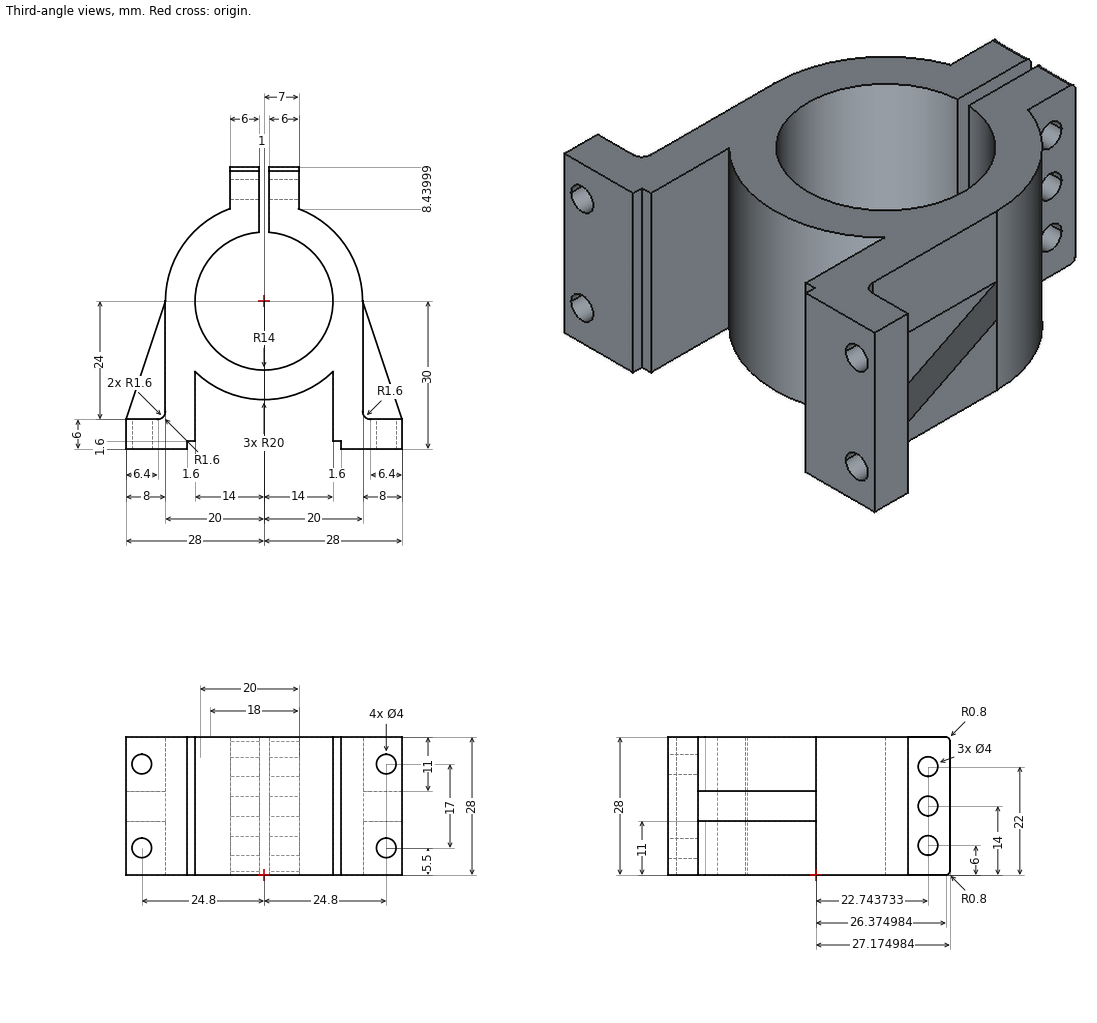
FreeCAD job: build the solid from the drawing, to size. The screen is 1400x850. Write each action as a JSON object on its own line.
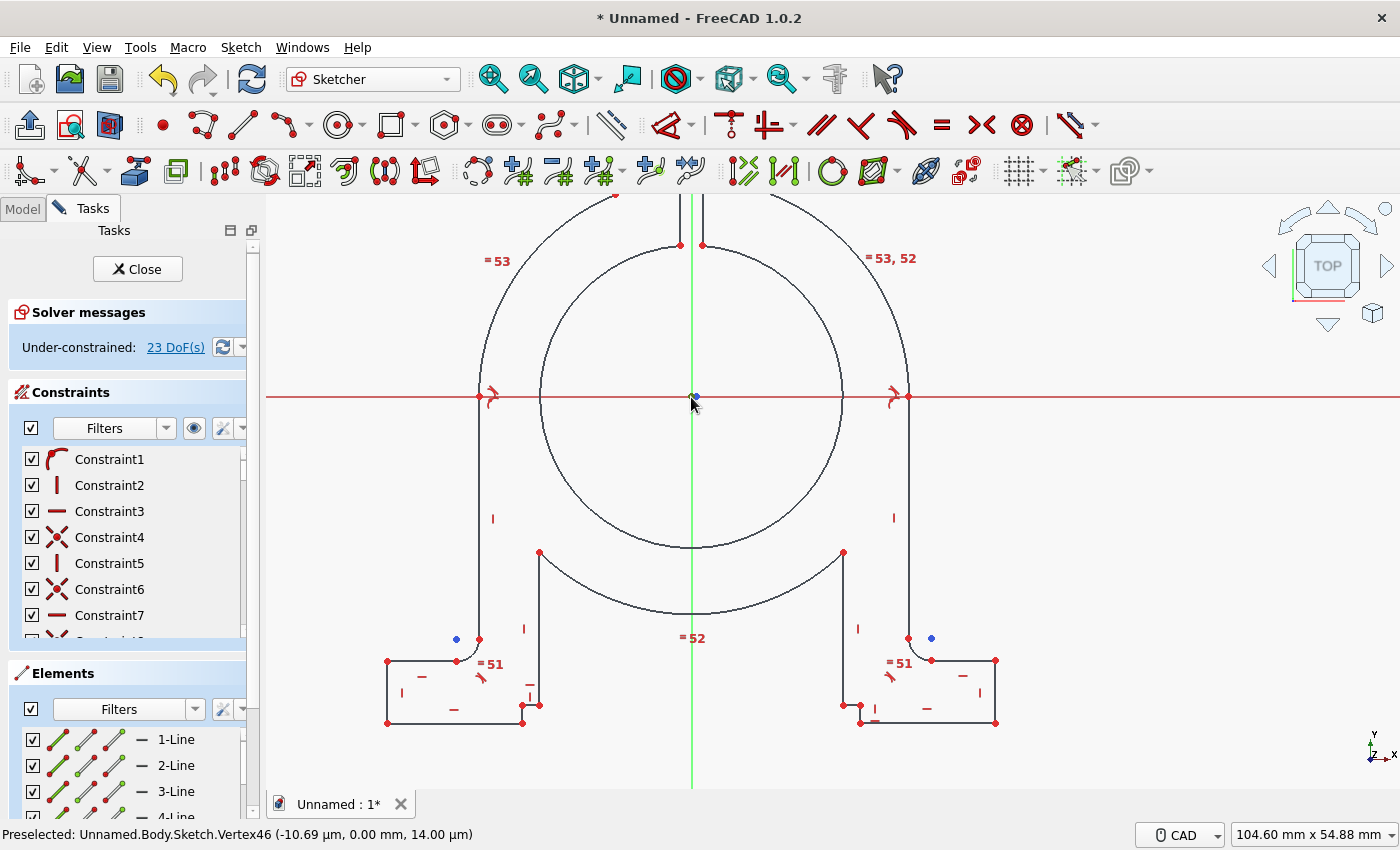
{"action": "left_click", "coordinate": [692, 722]}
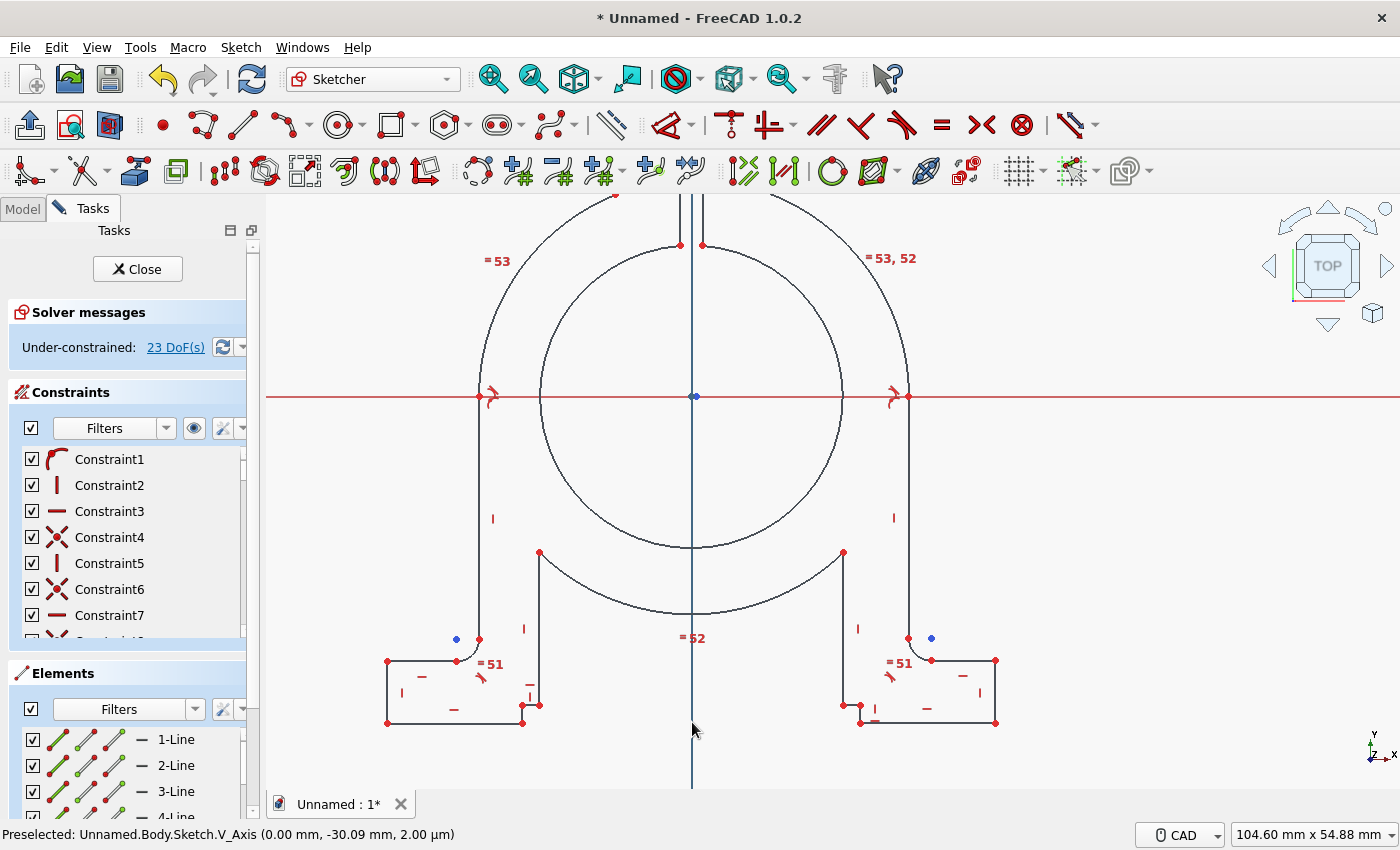
{"action": "left_click", "coordinate": [730, 126]}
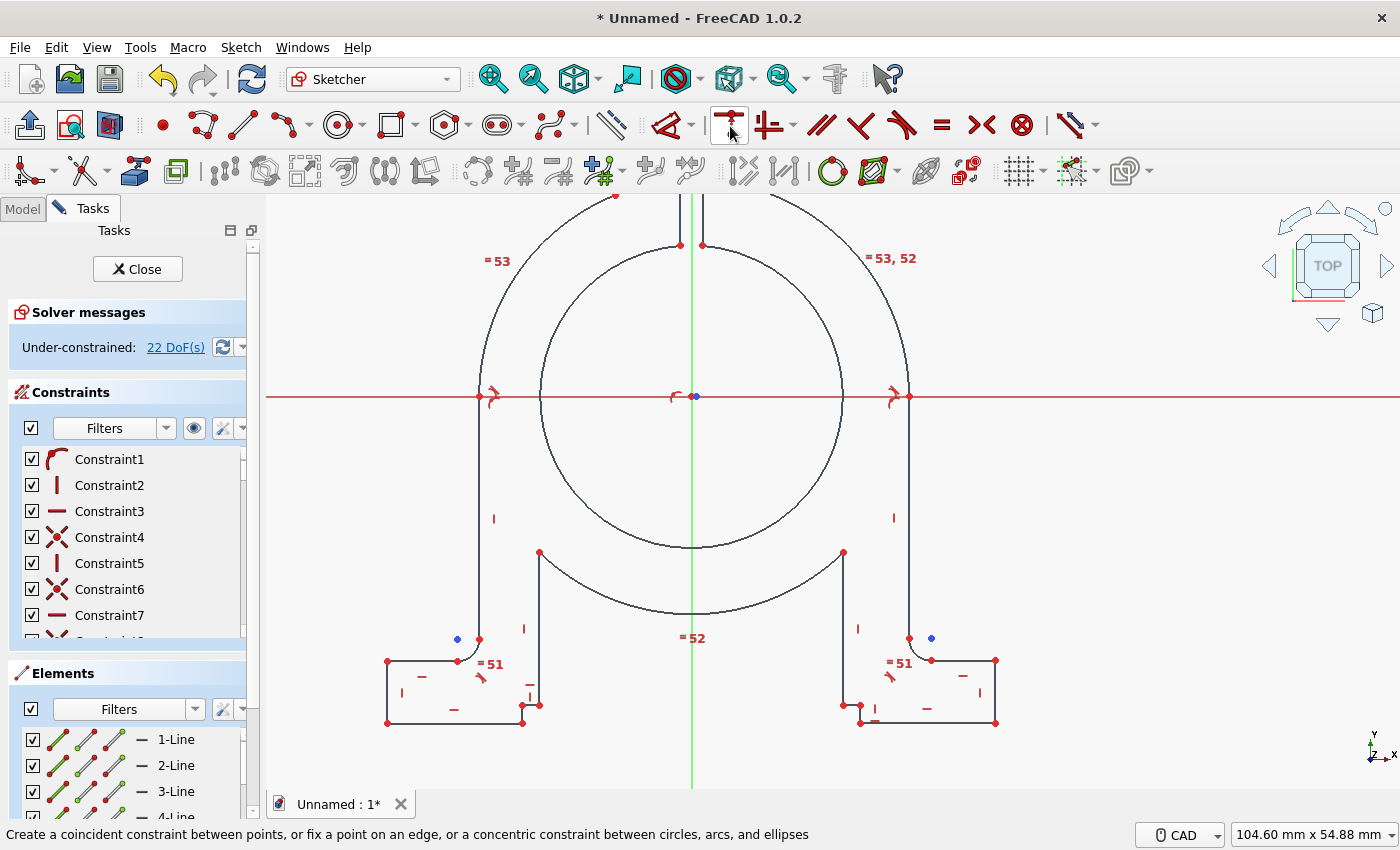
{"action": "left_click", "coordinate": [697, 397]}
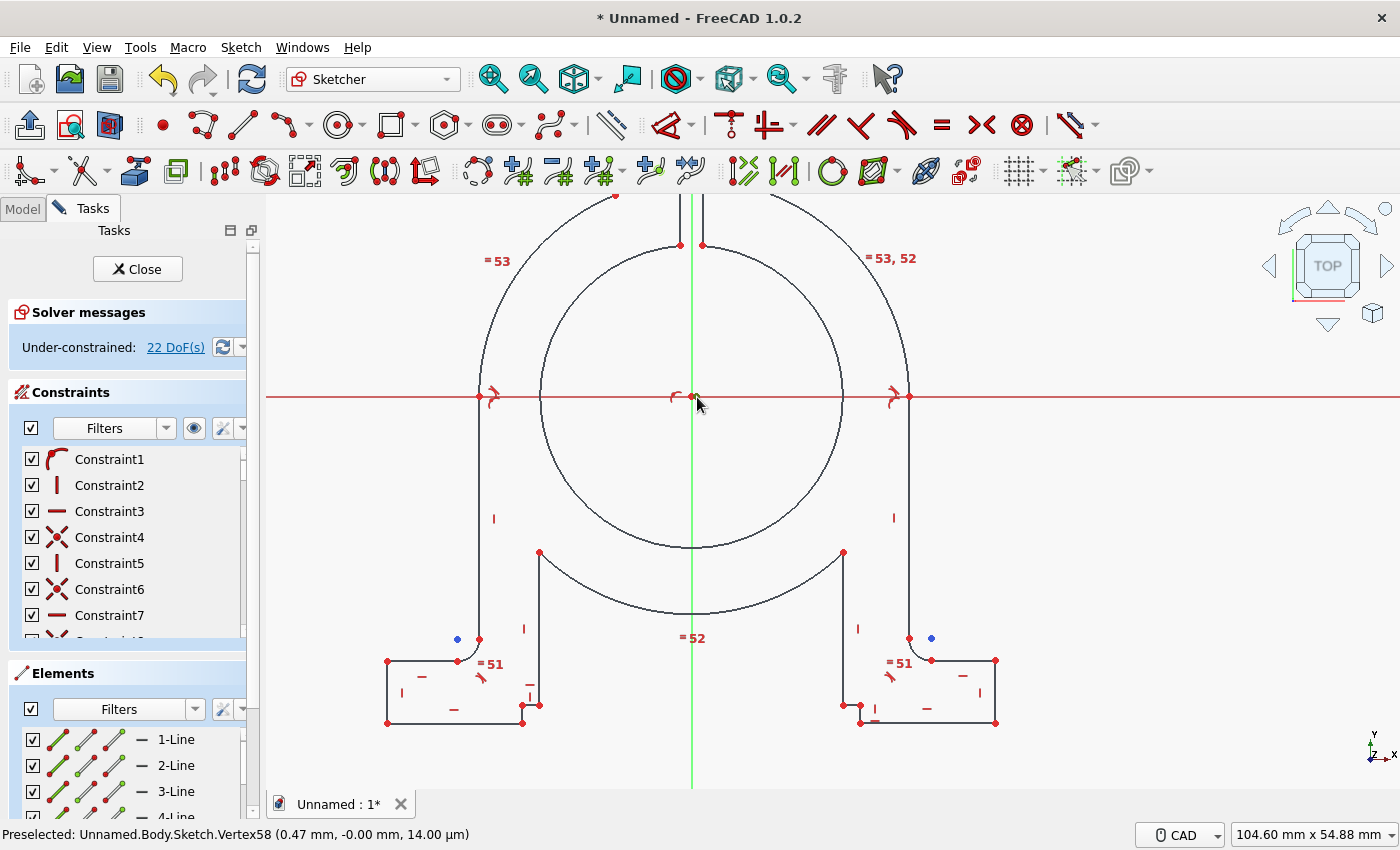
{"action": "left_click", "coordinate": [692, 722]}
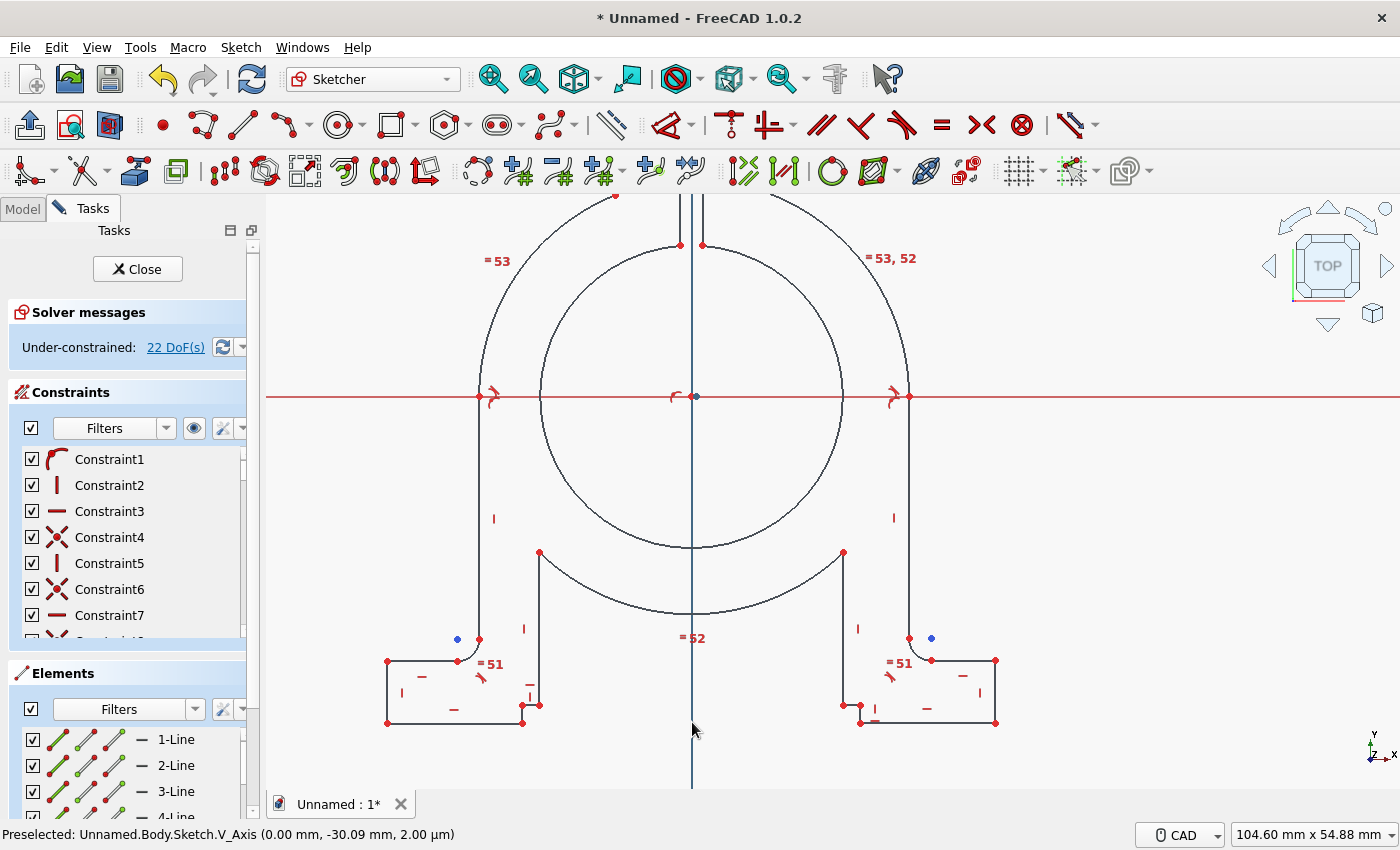
{"action": "left_click", "coordinate": [730, 126]}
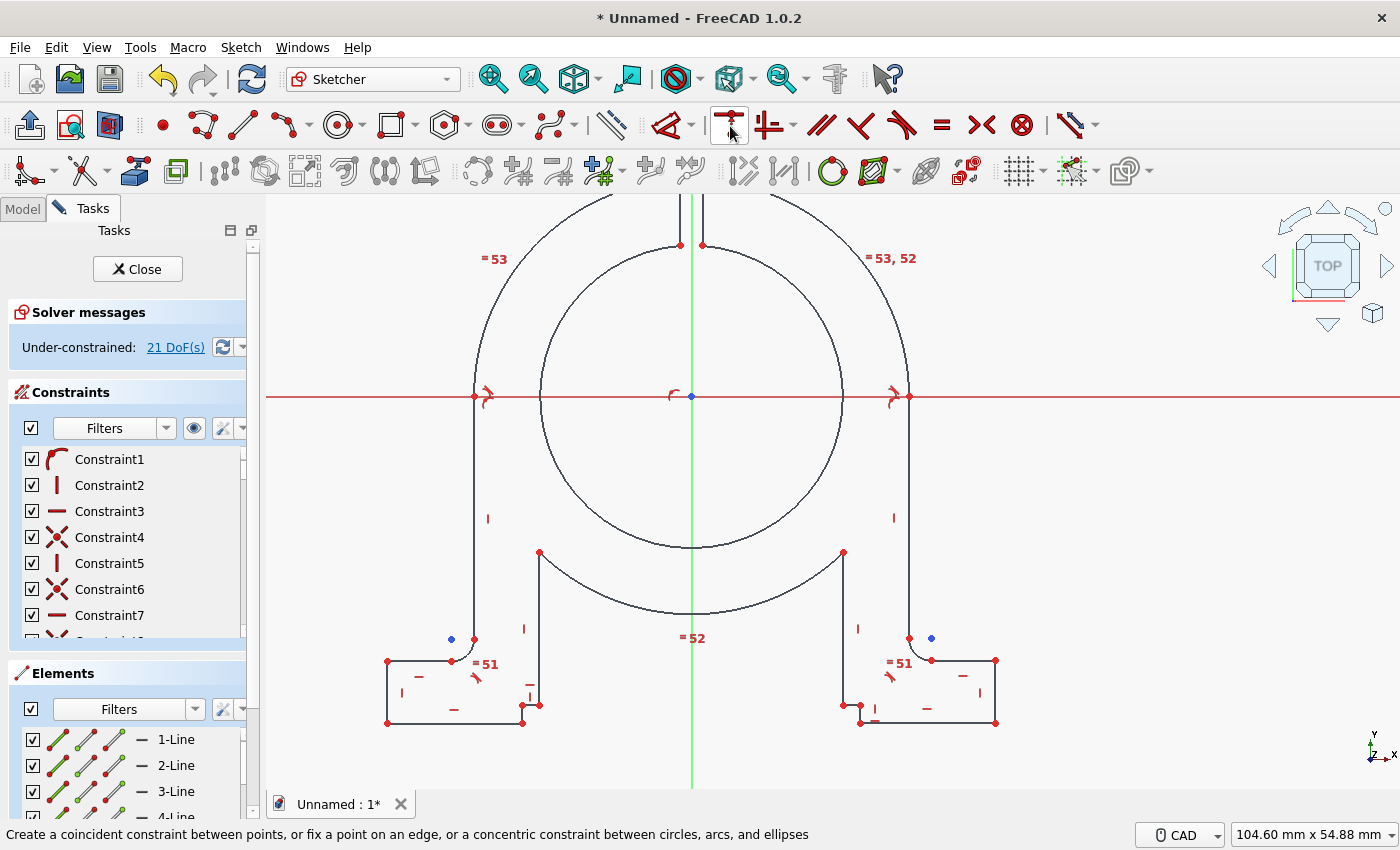
{"action": "left_click", "coordinate": [666, 126]}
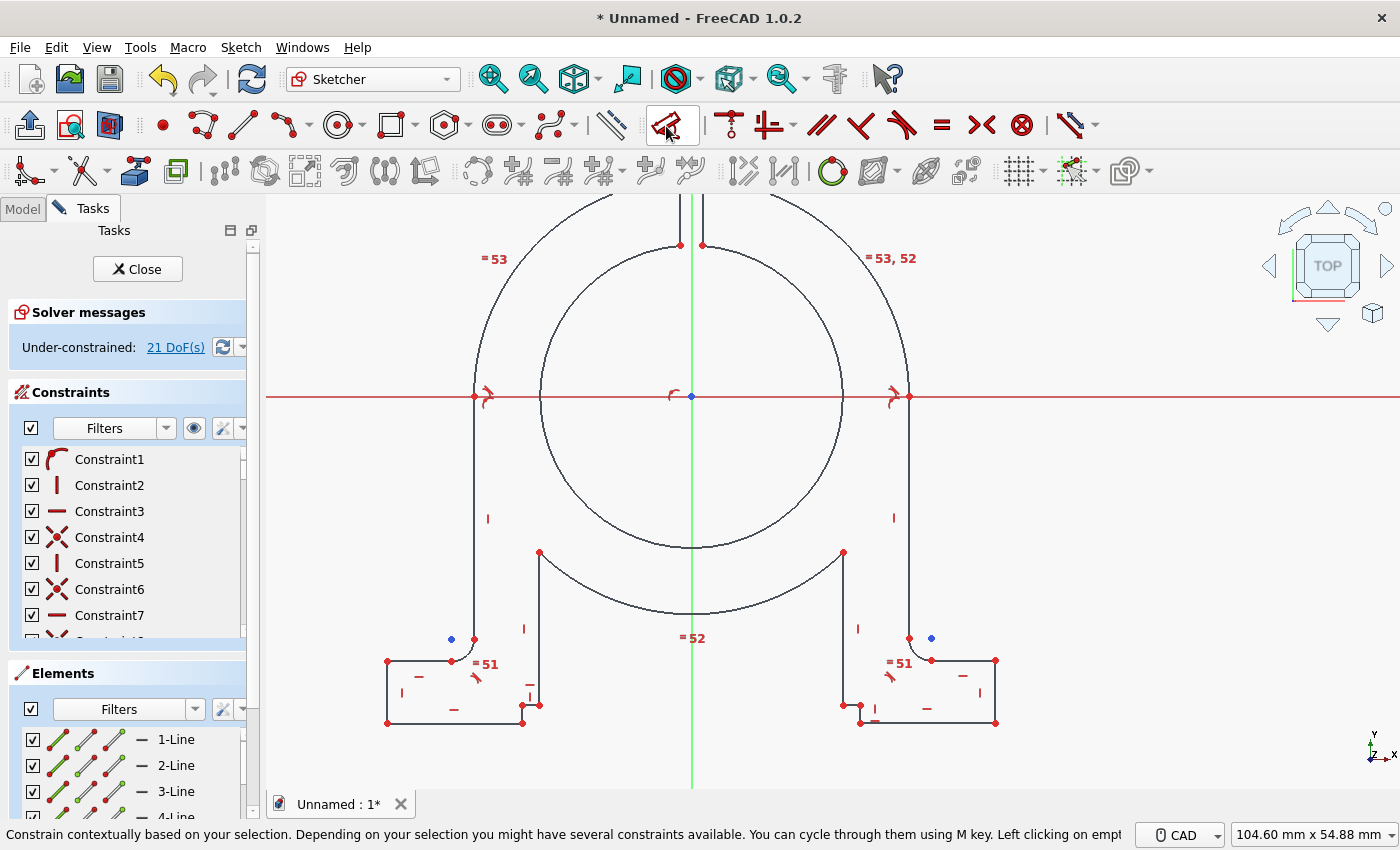
{"action": "scroll", "coordinate": [462, 659], "scroll_direction": "up", "scroll_amount": 5}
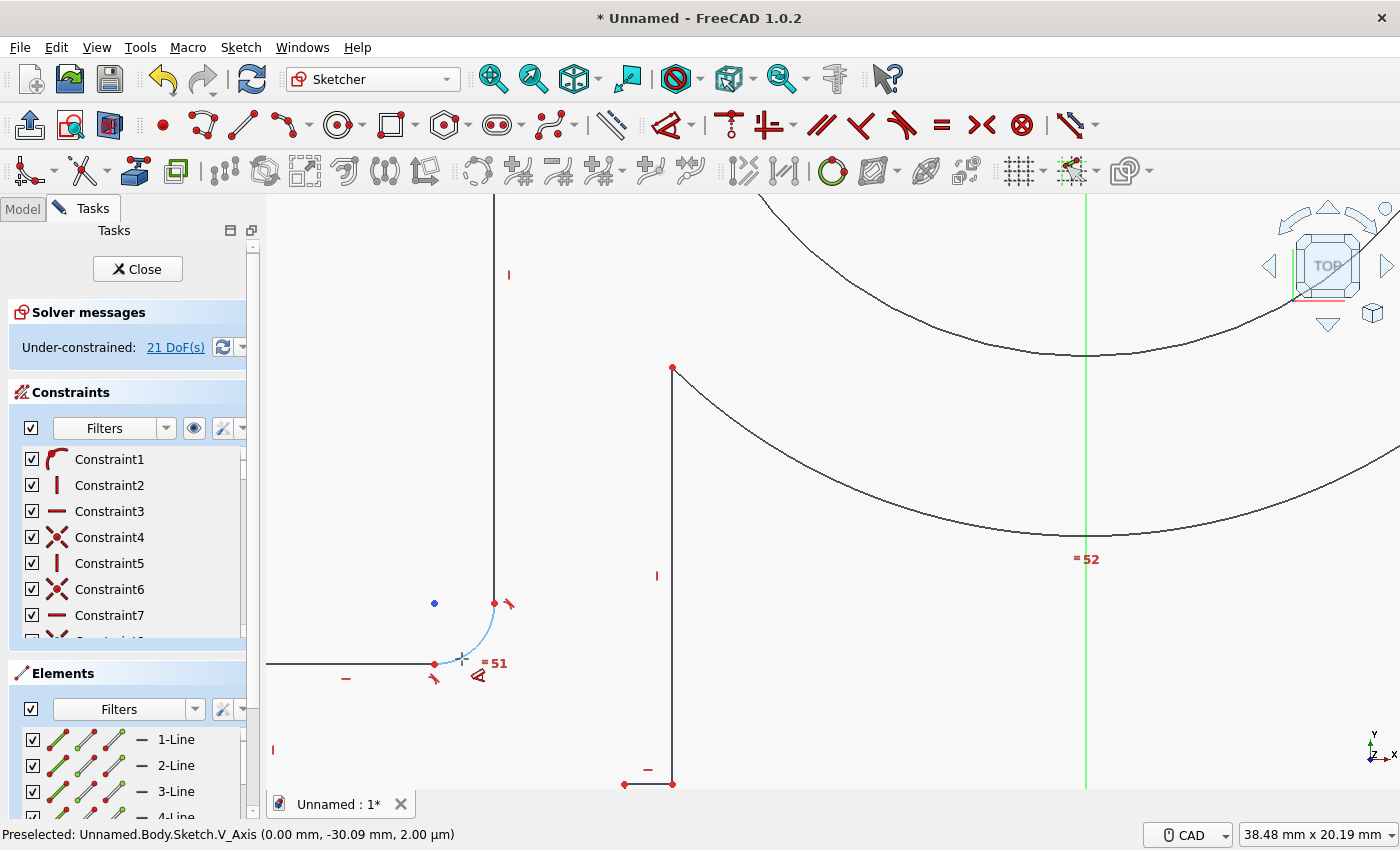
{"action": "left_click", "coordinate": [462, 657]}
{"action": "left_click", "coordinate": [477, 685]}